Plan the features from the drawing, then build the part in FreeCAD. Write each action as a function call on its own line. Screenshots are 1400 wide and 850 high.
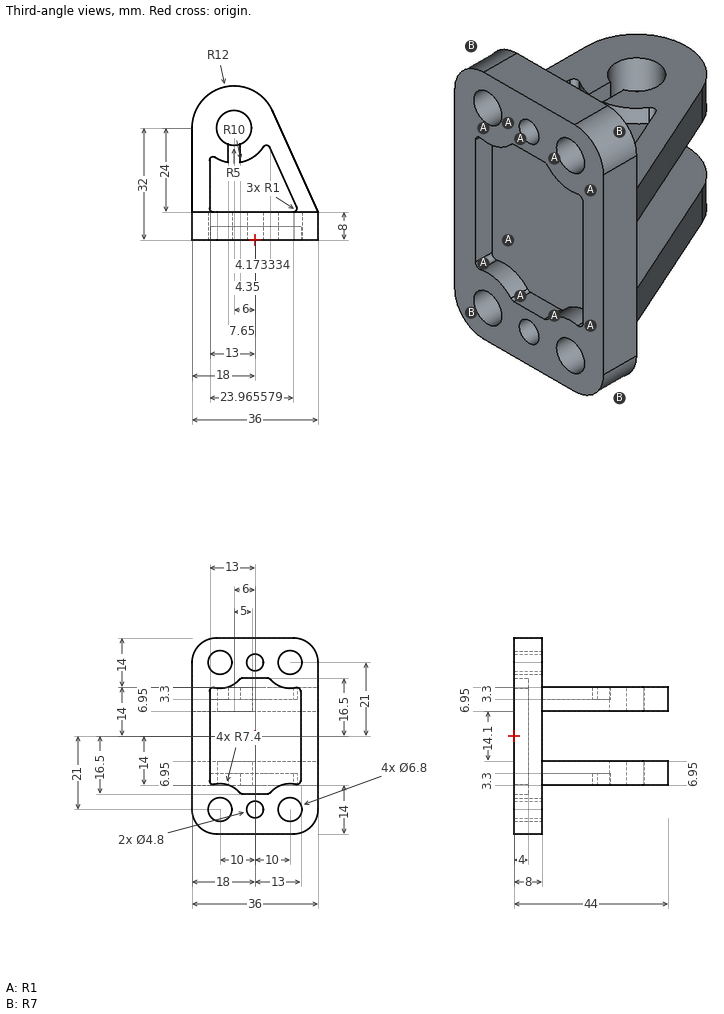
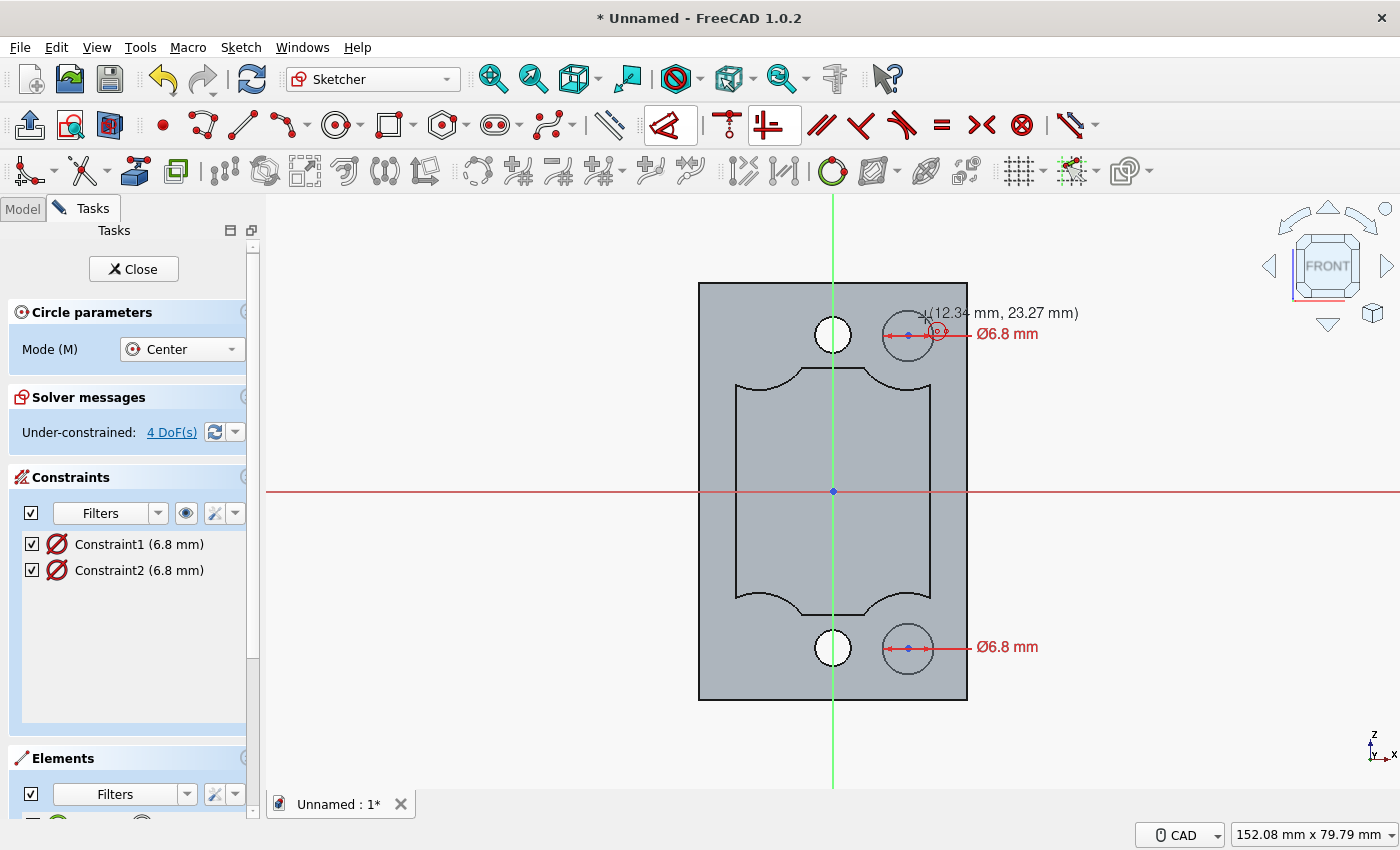
click(758, 648)
move(776, 630)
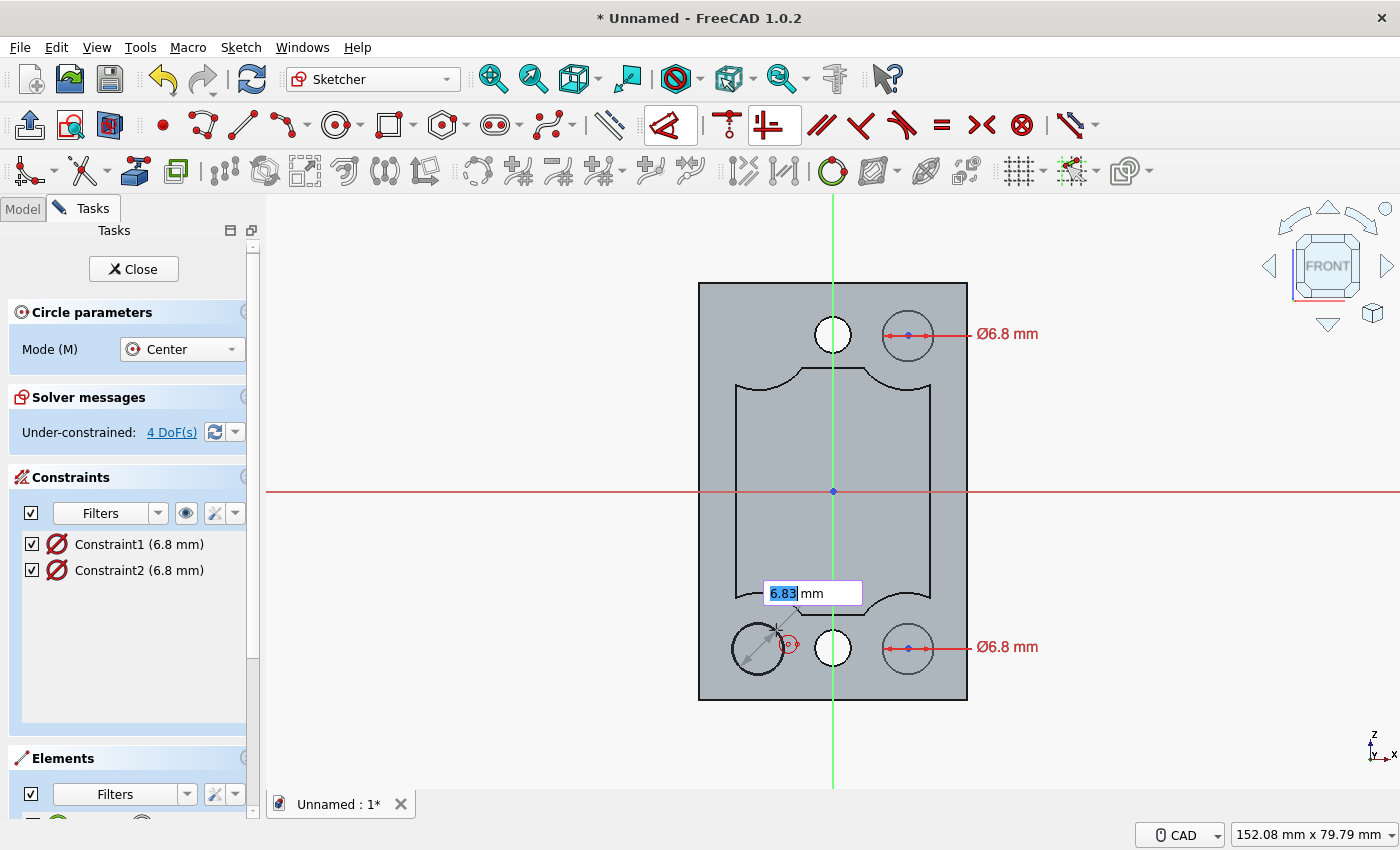
text(6.8)
key(Return)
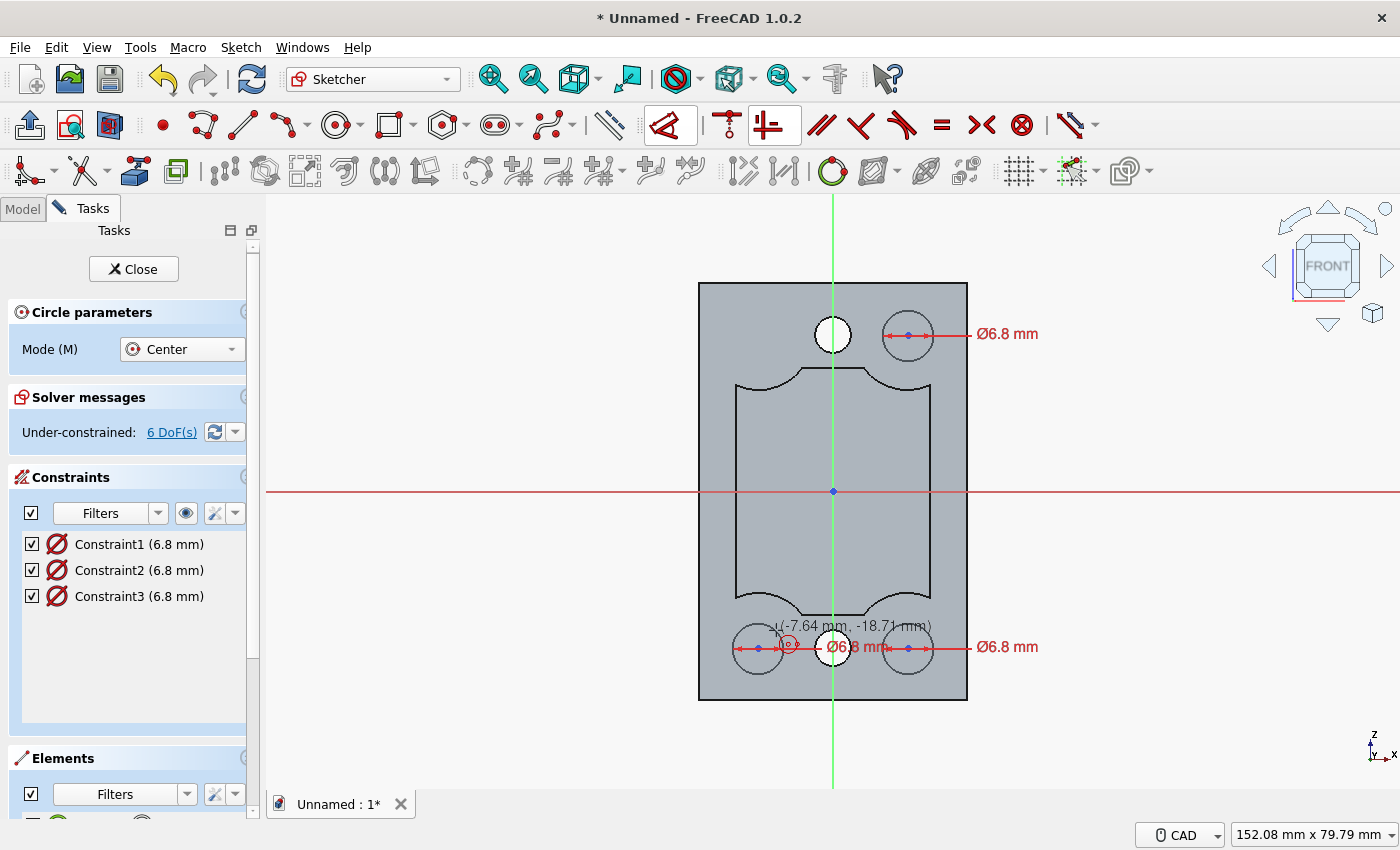
click(758, 335)
move(776, 317)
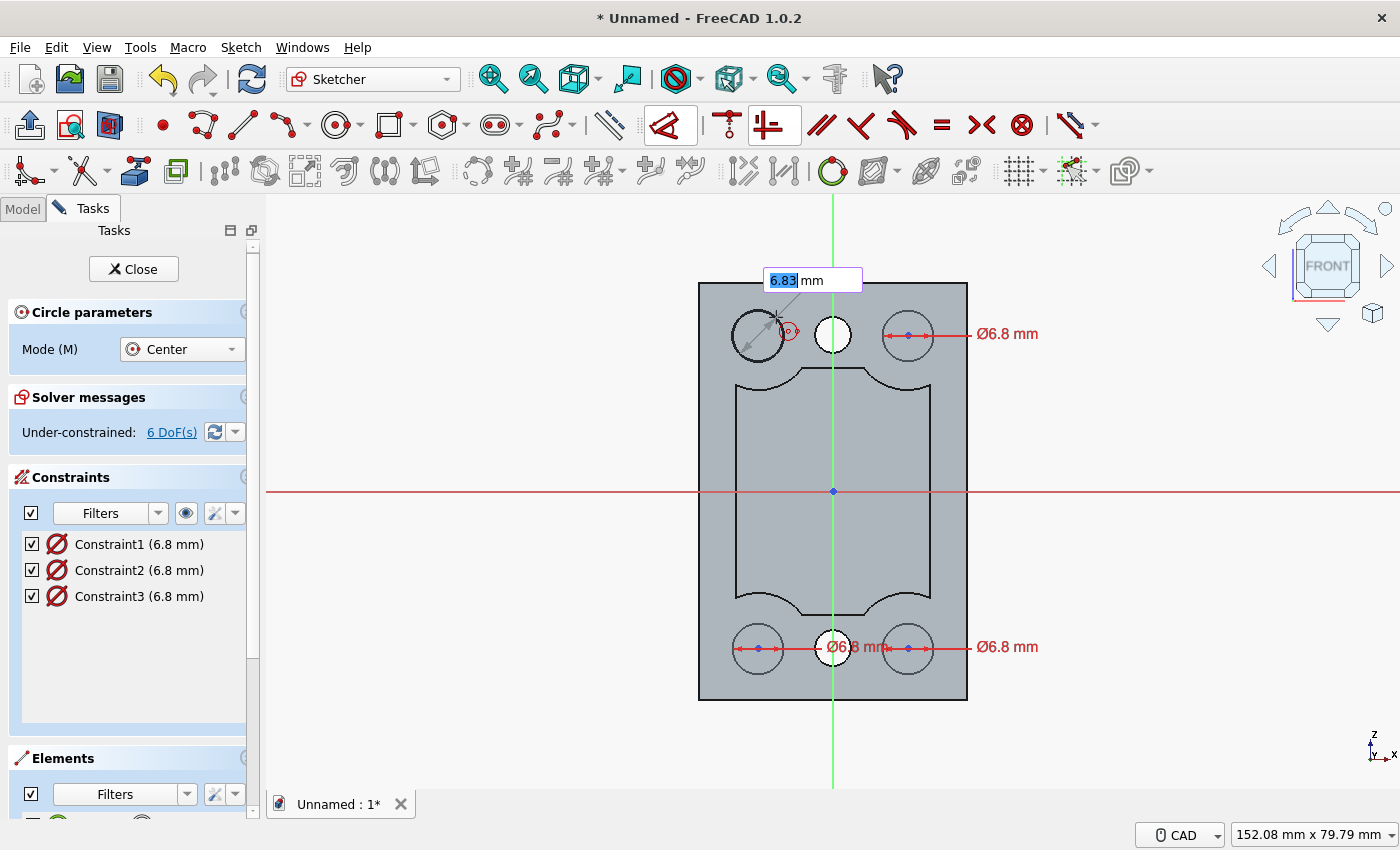
text(6.8)
key(Return)
key(Escape)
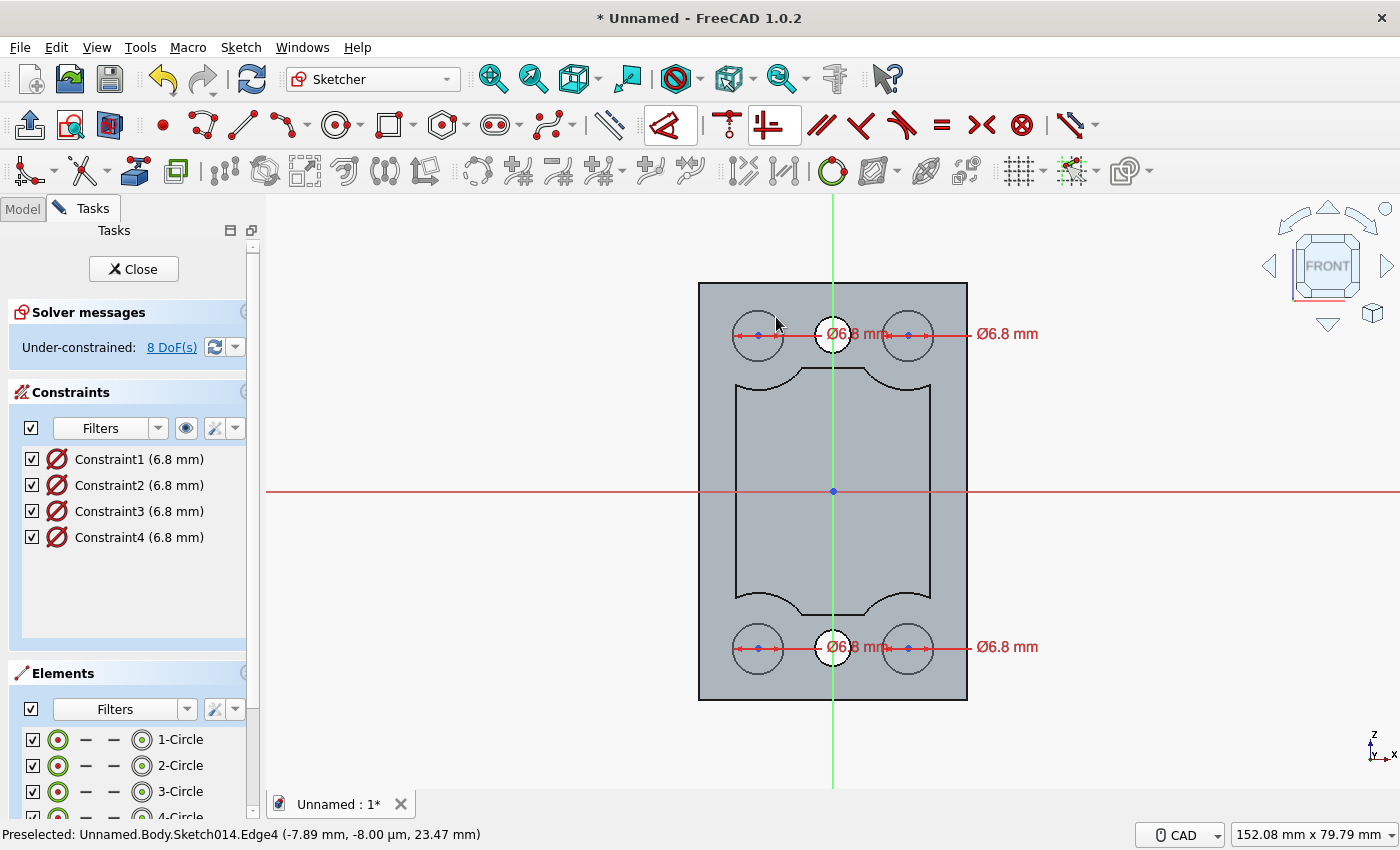
click(908, 649)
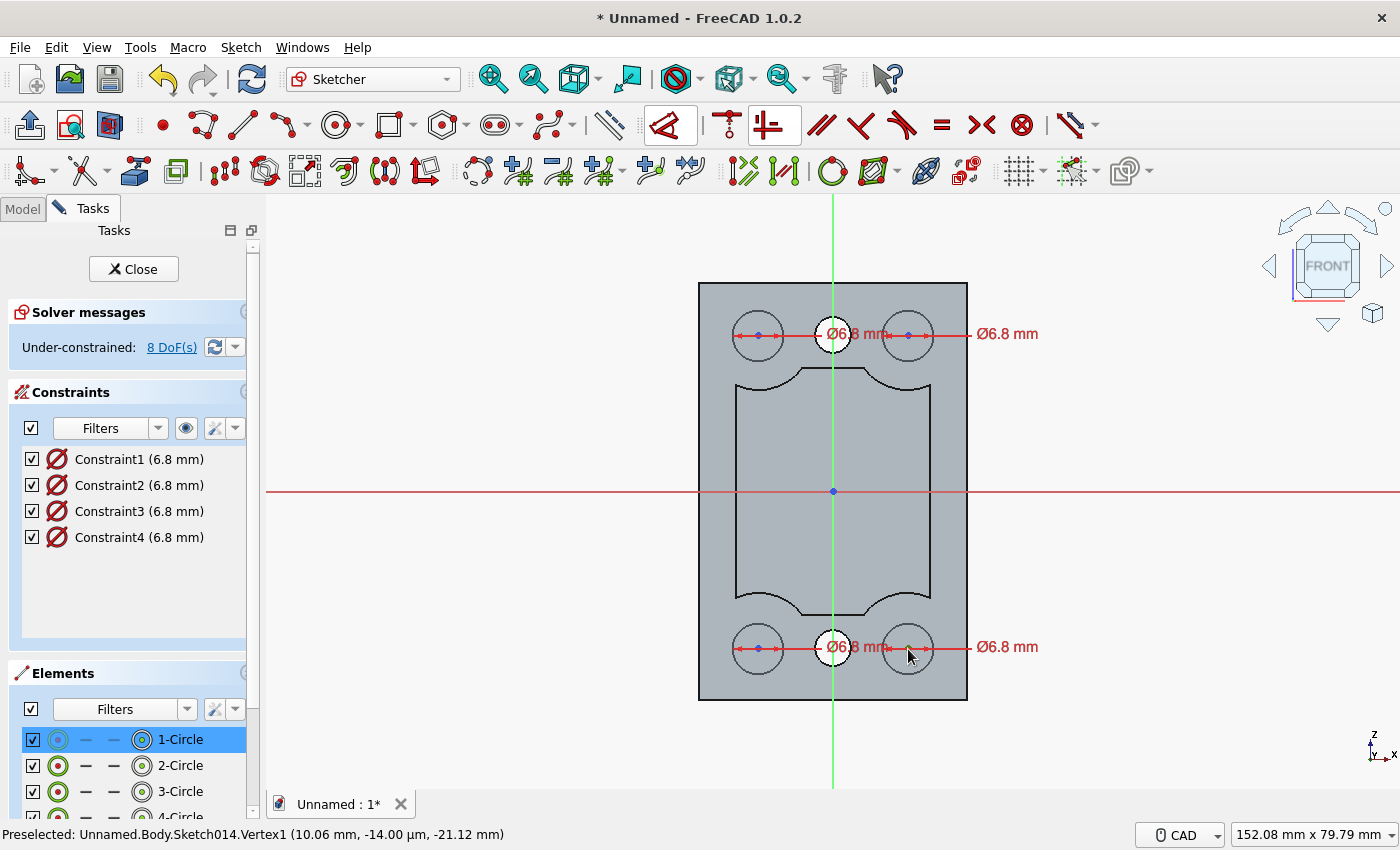
click(908, 336)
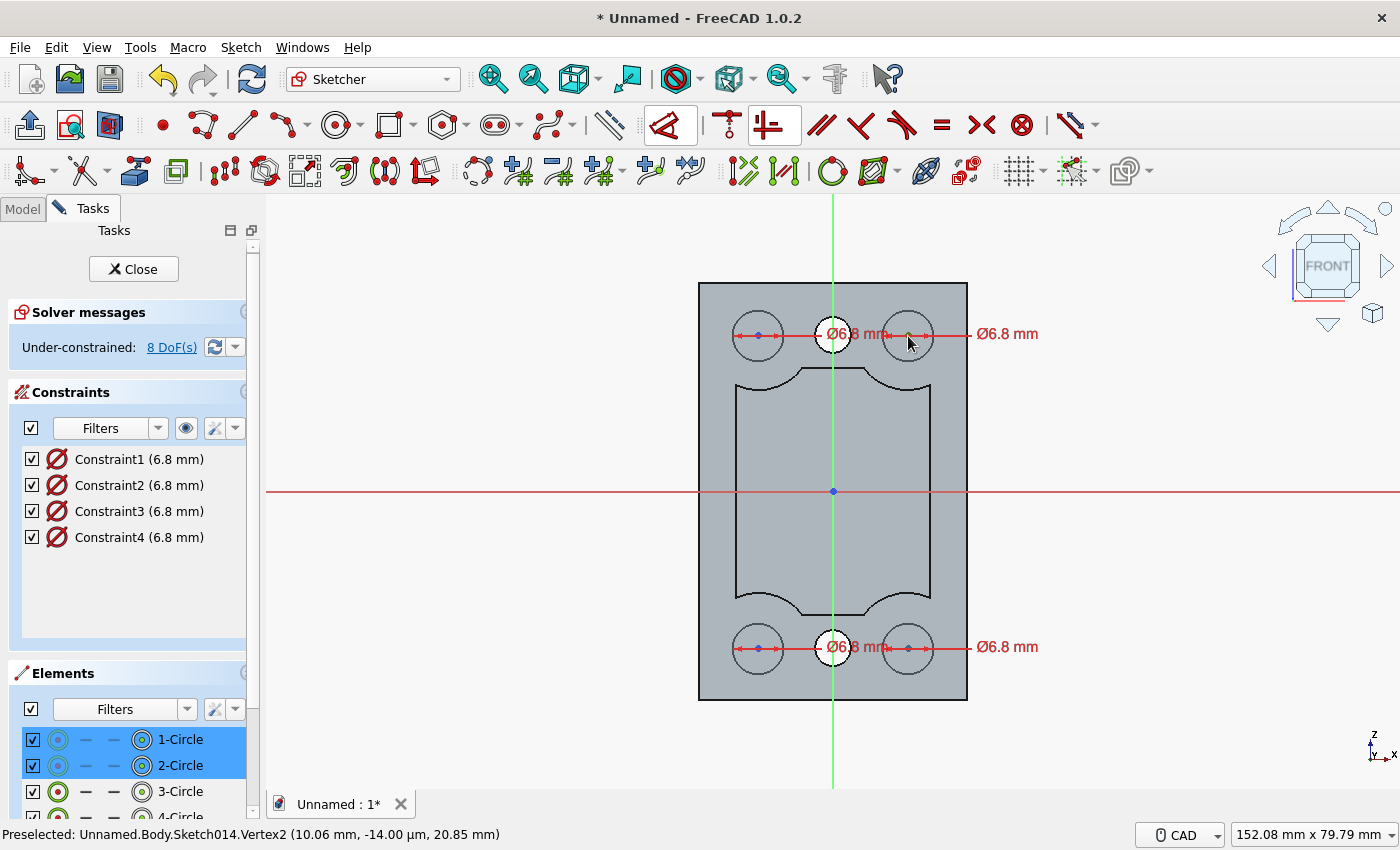
key(v)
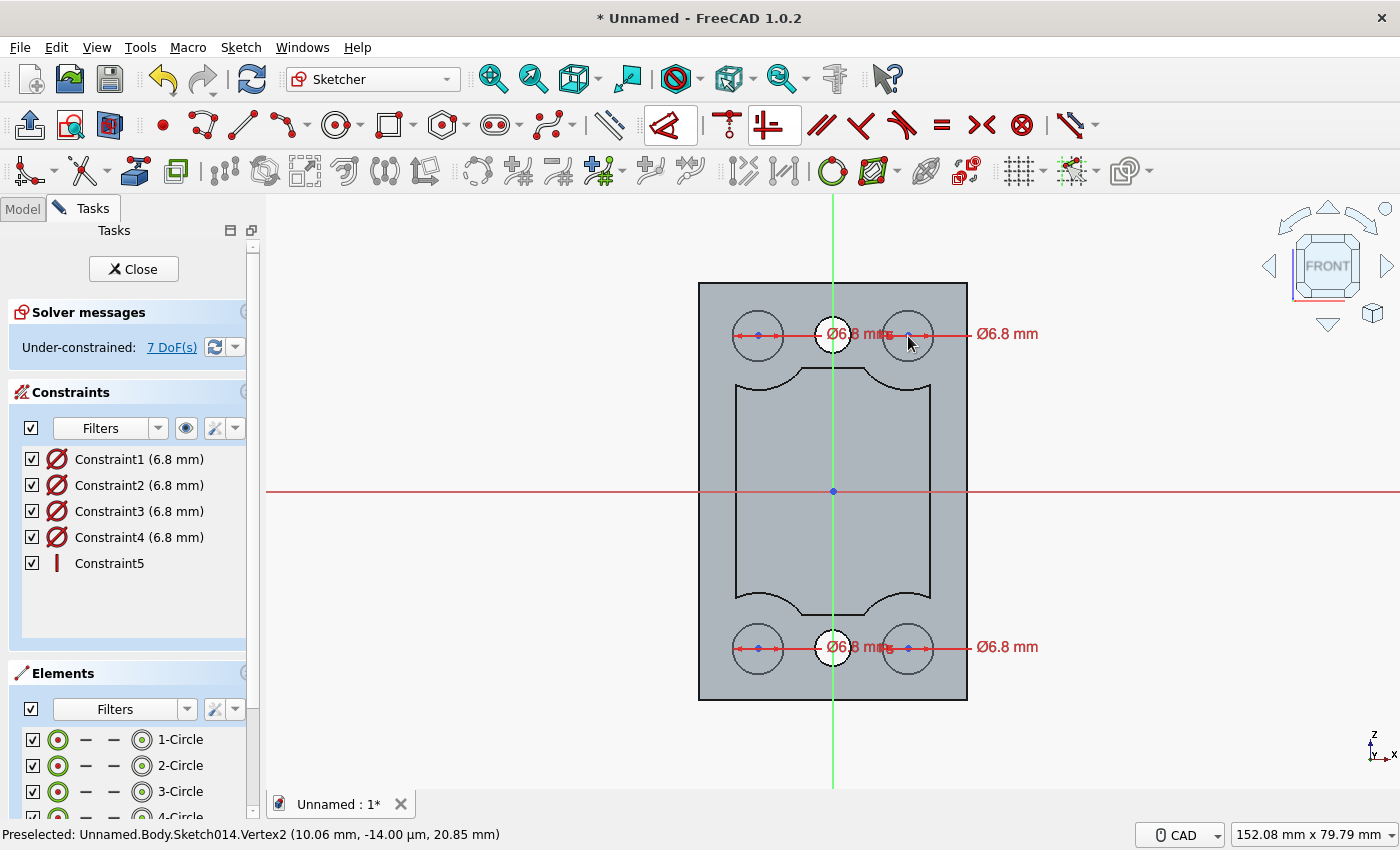
click(908, 649)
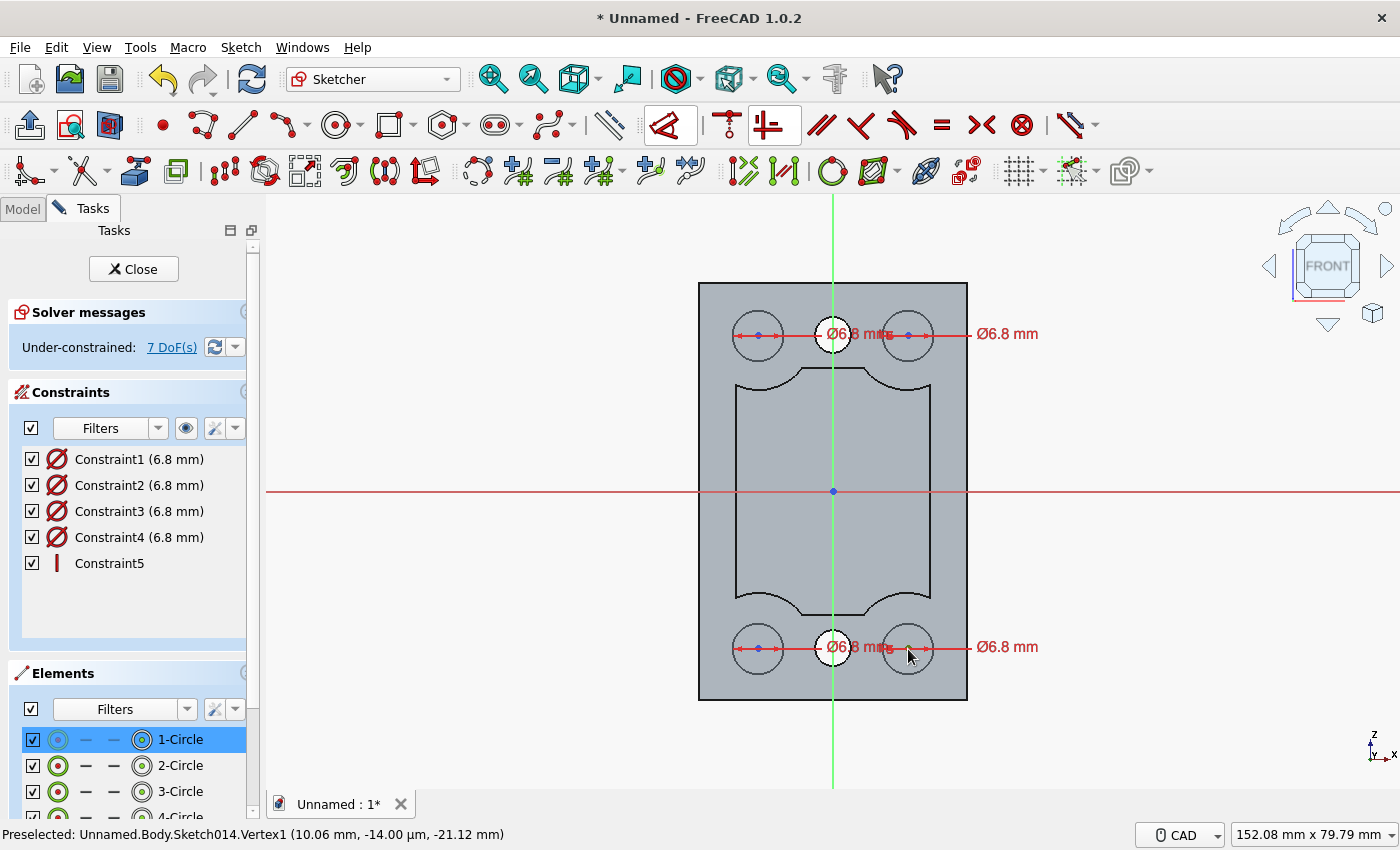
click(758, 649)